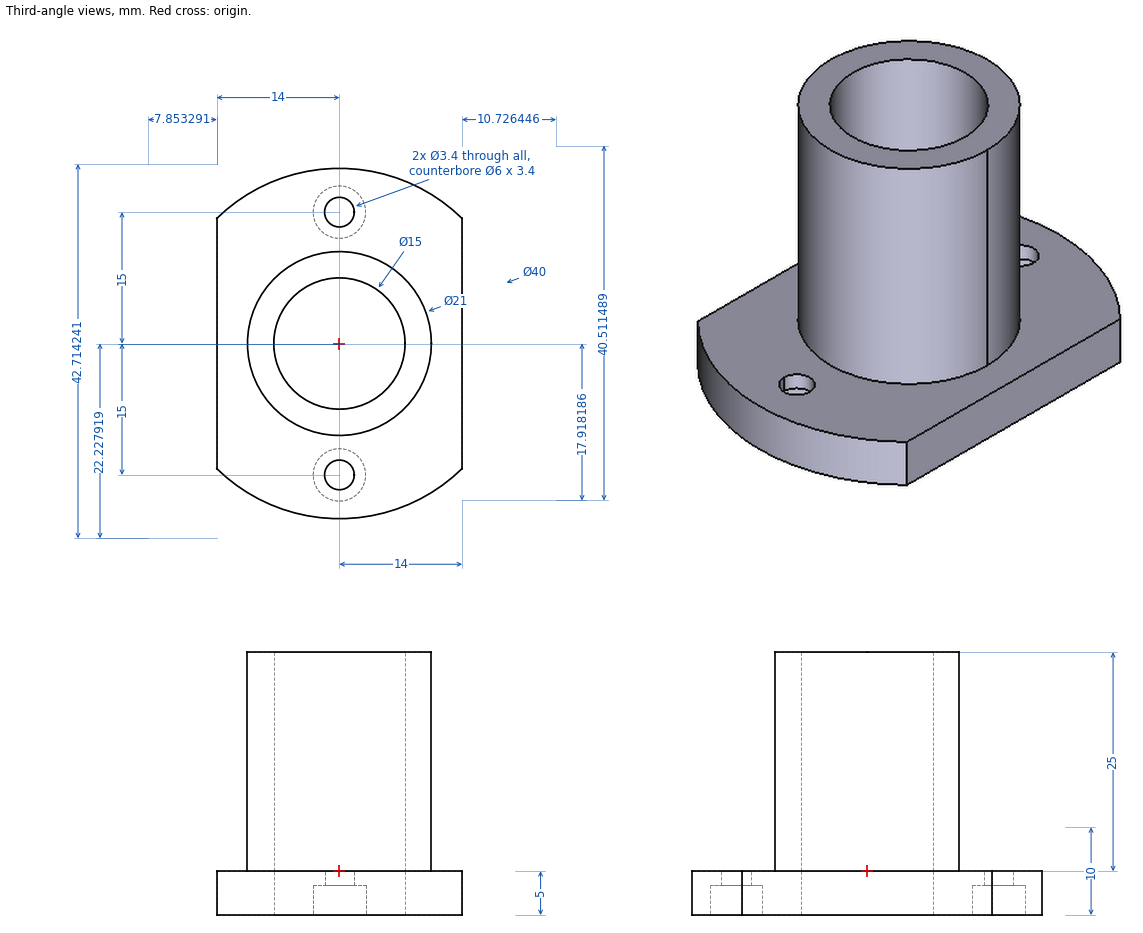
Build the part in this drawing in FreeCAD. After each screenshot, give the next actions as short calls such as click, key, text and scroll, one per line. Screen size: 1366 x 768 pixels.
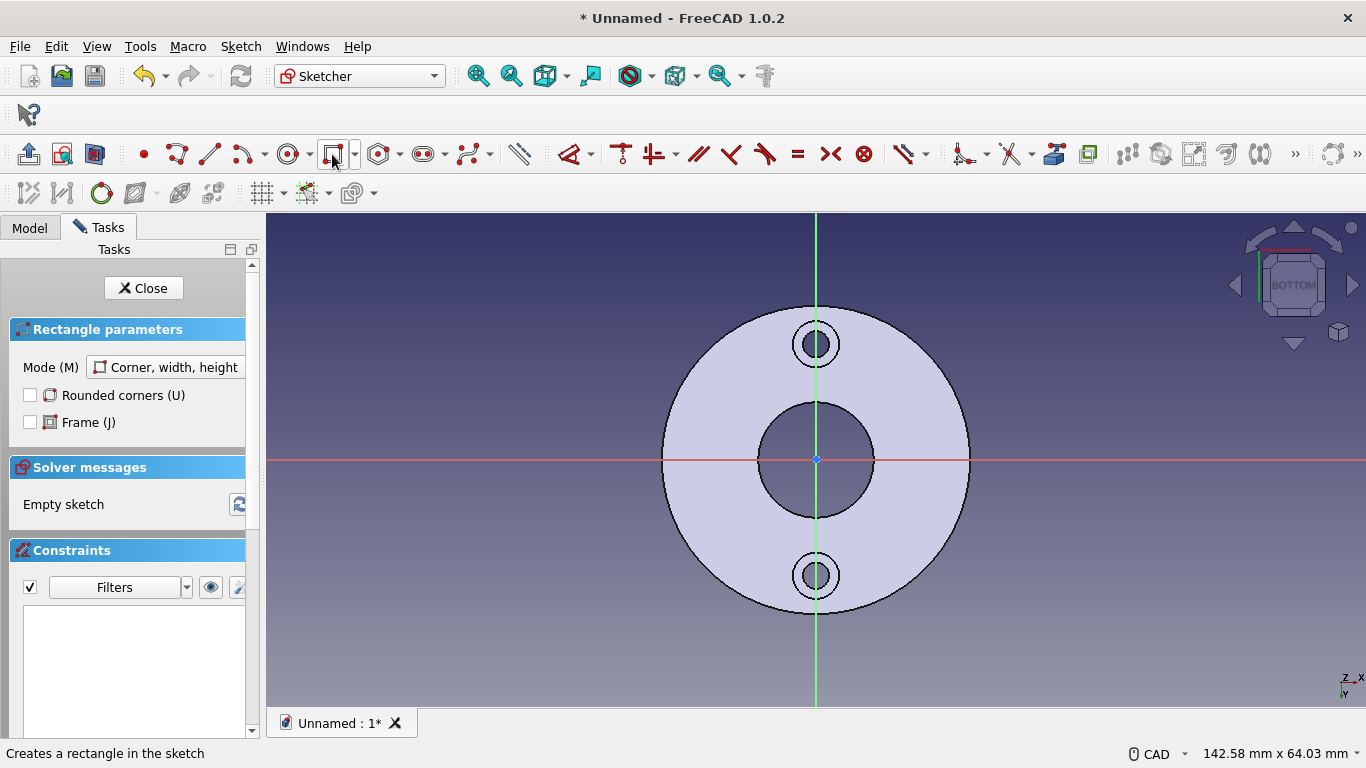
click(924, 322)
move(1007, 634)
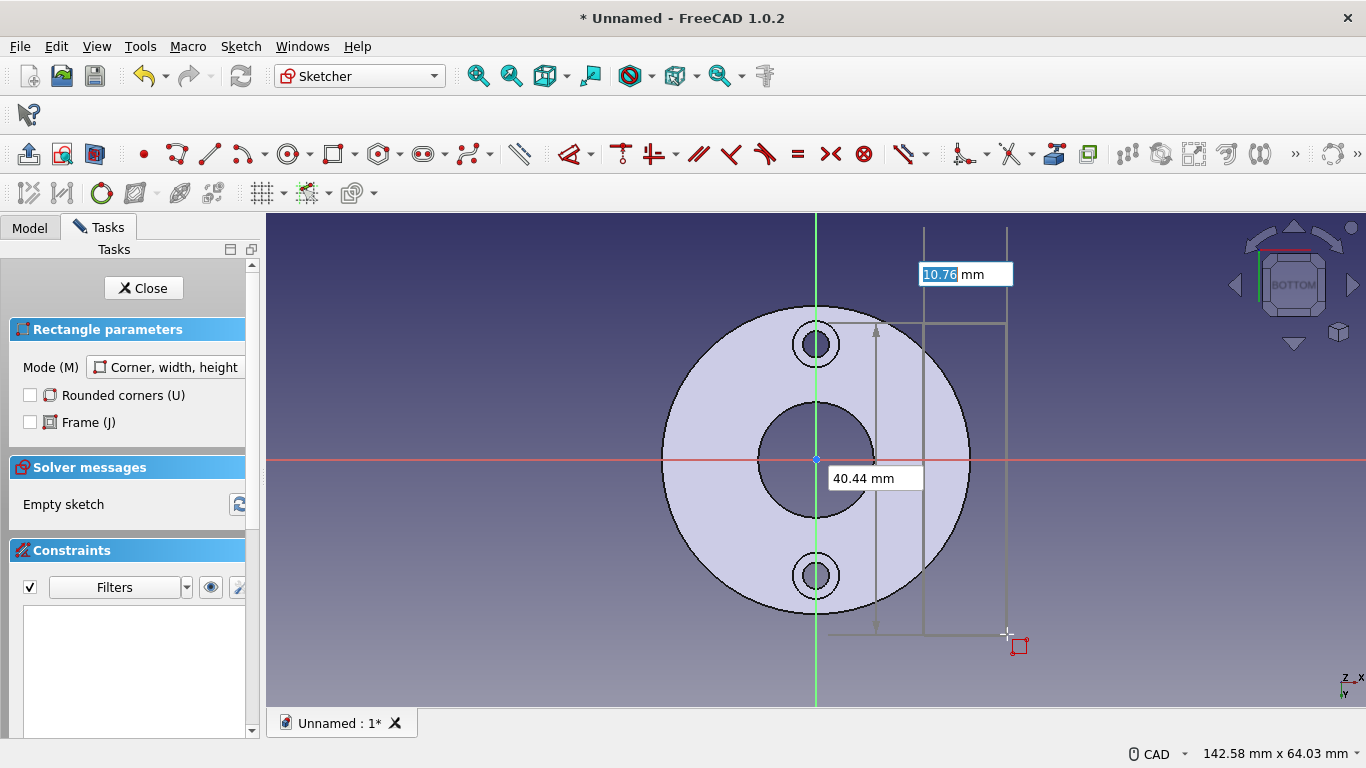
text(10.726446)
key(Tab)
text(40.511489)
key(Return)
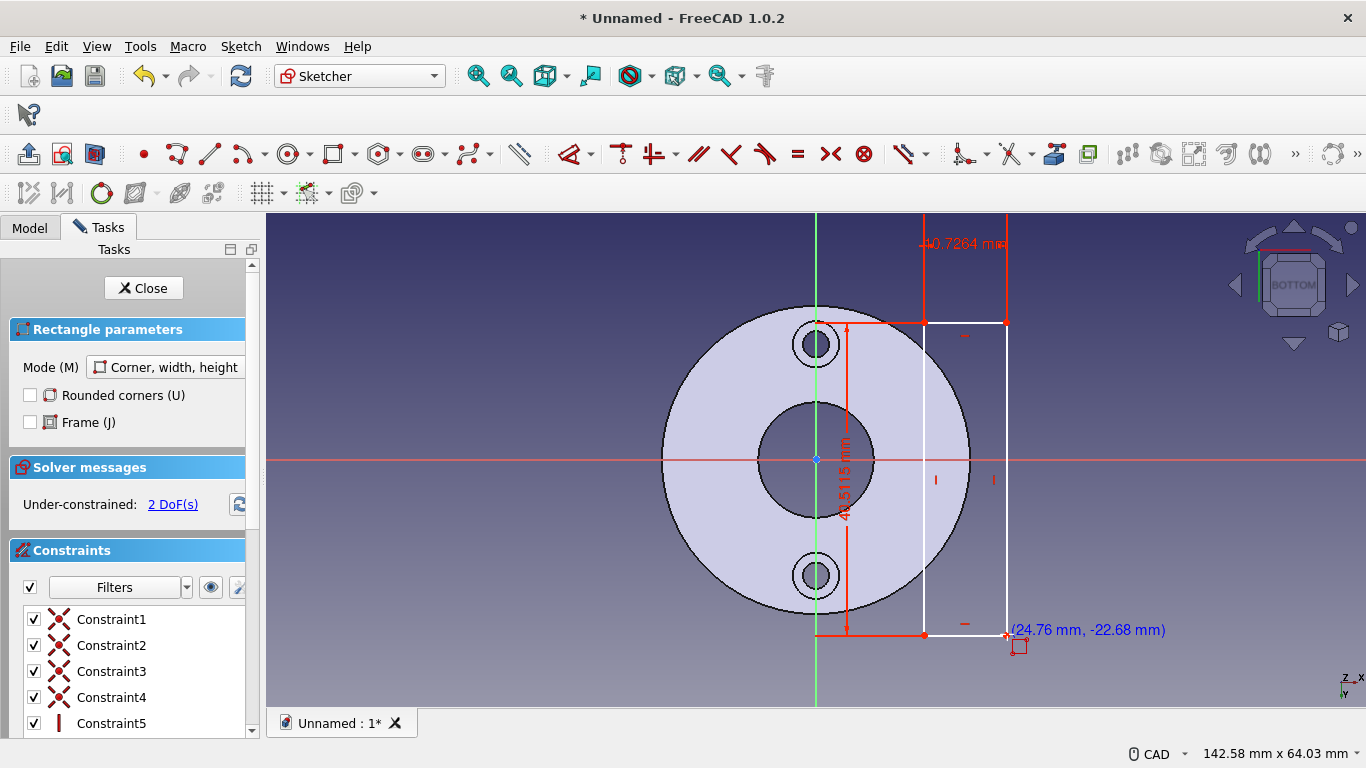
click(647, 289)
move(708, 618)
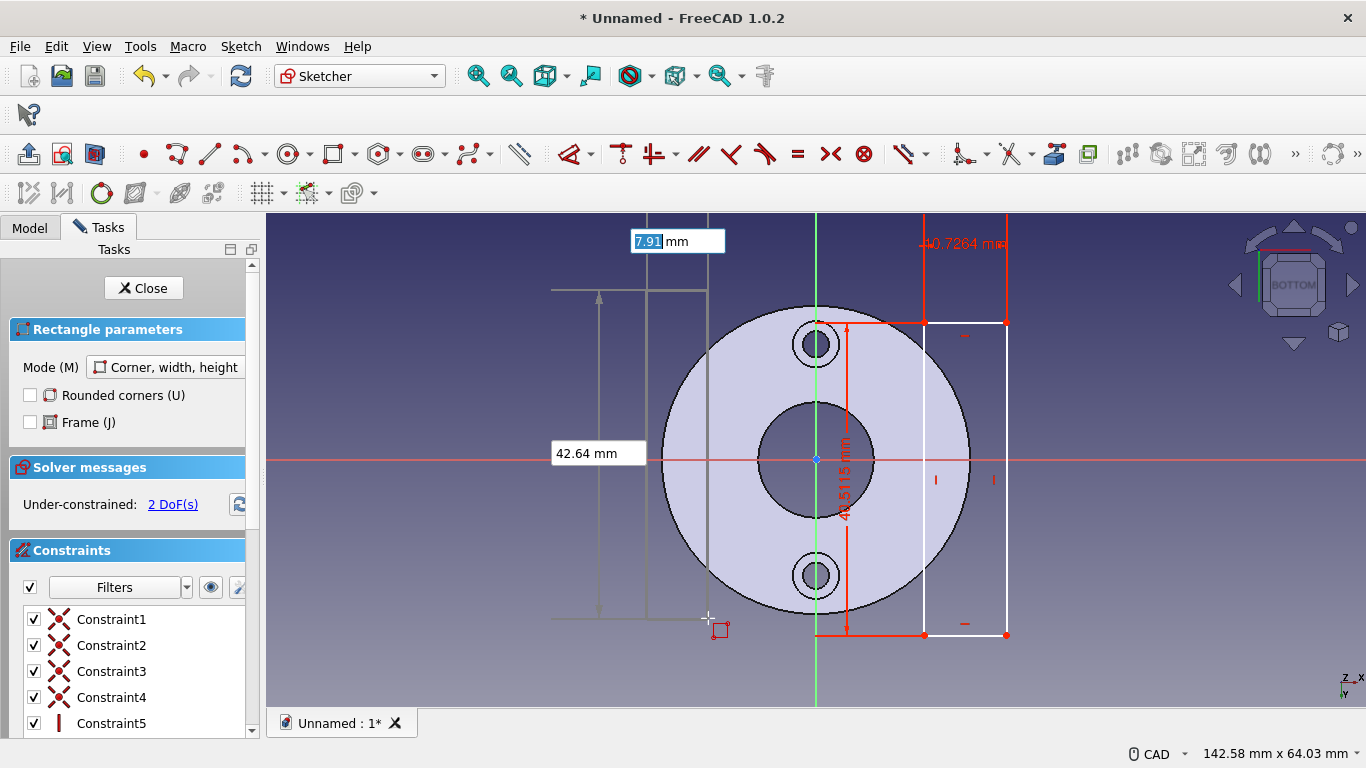
text(7.853291)
key(Tab)
text(42.714241)
key(Return)
key(Escape)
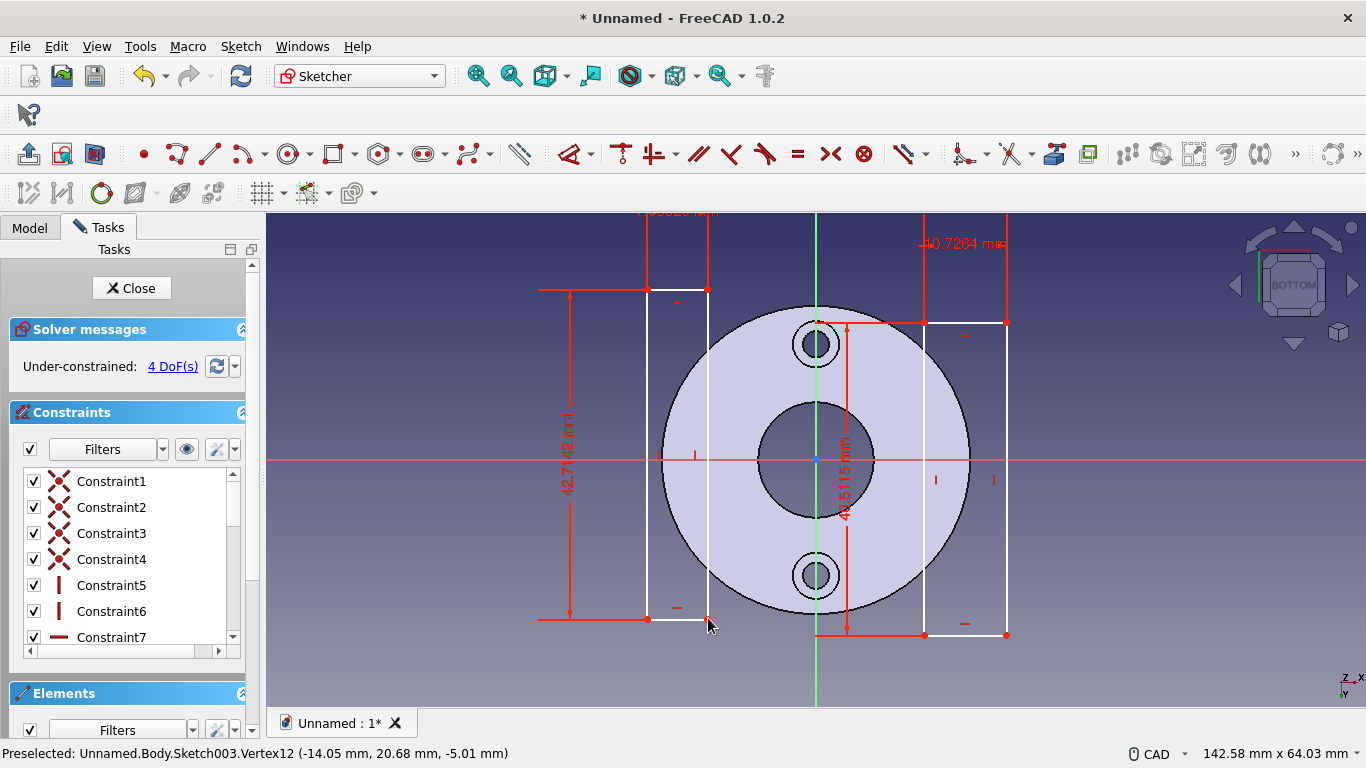
click(568, 154)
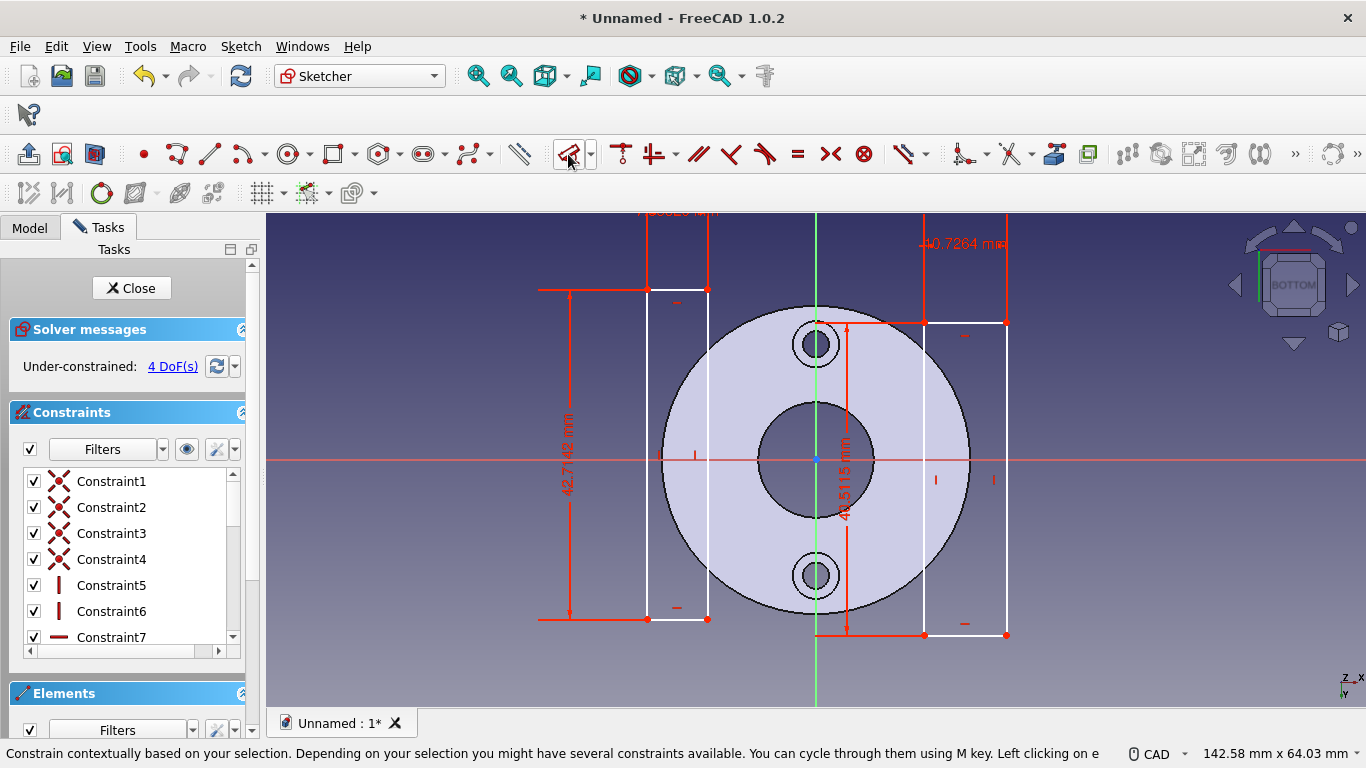
click(924, 323)
click(870, 289)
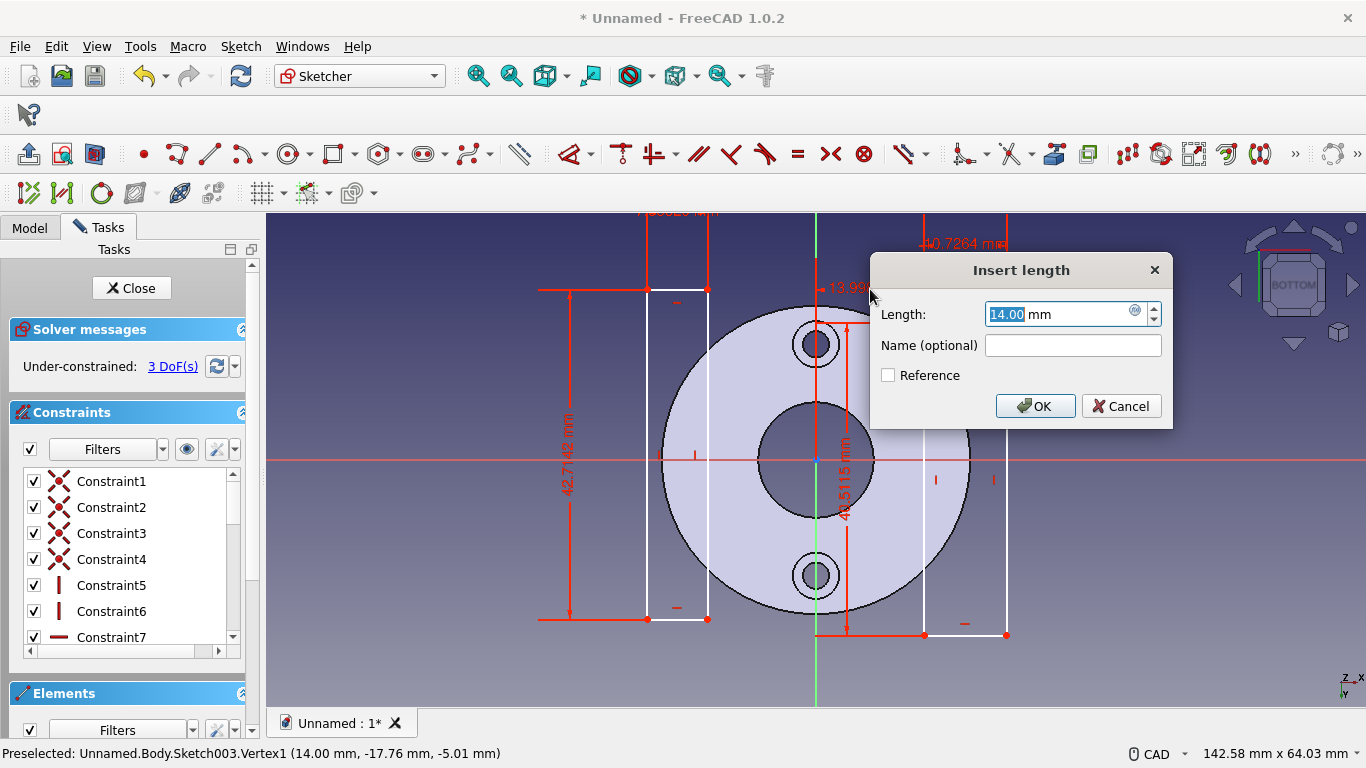
text(14)
key(Return)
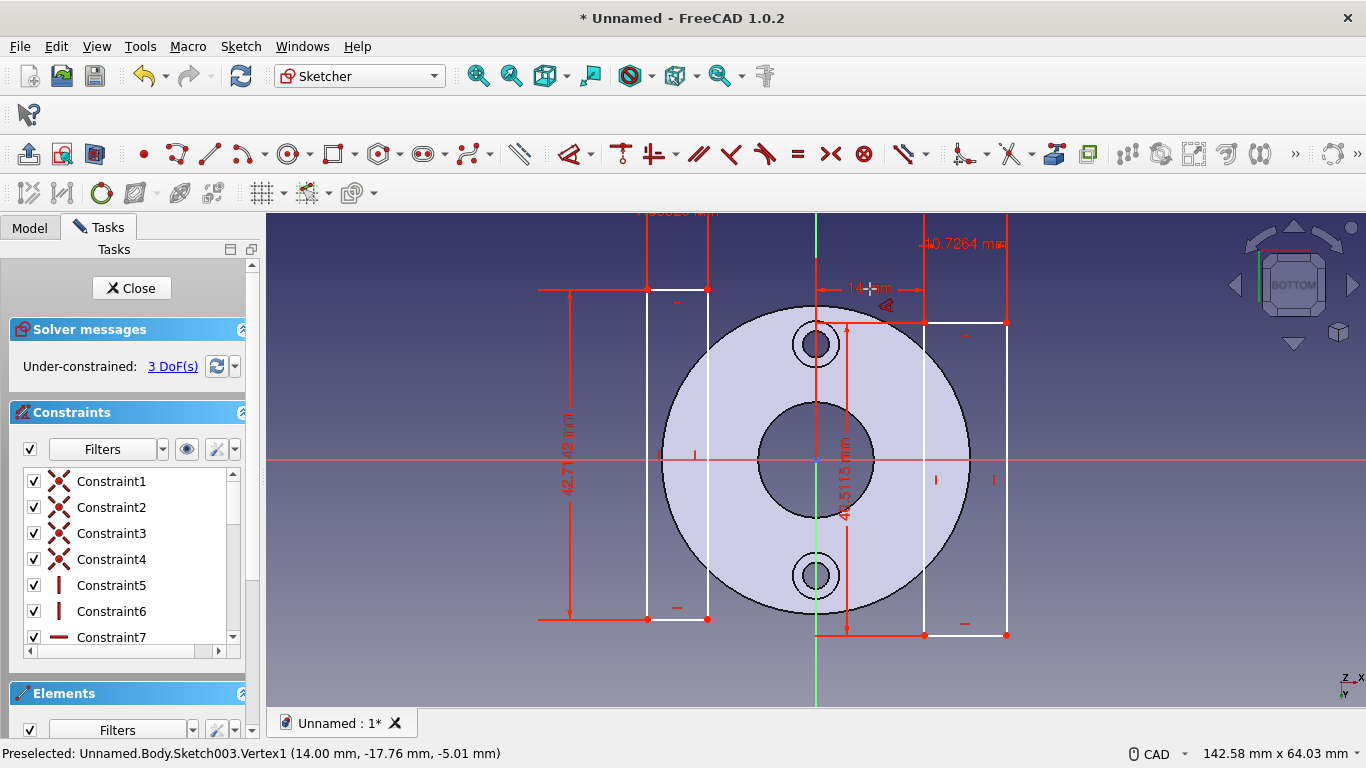
click(708, 620)
click(762, 654)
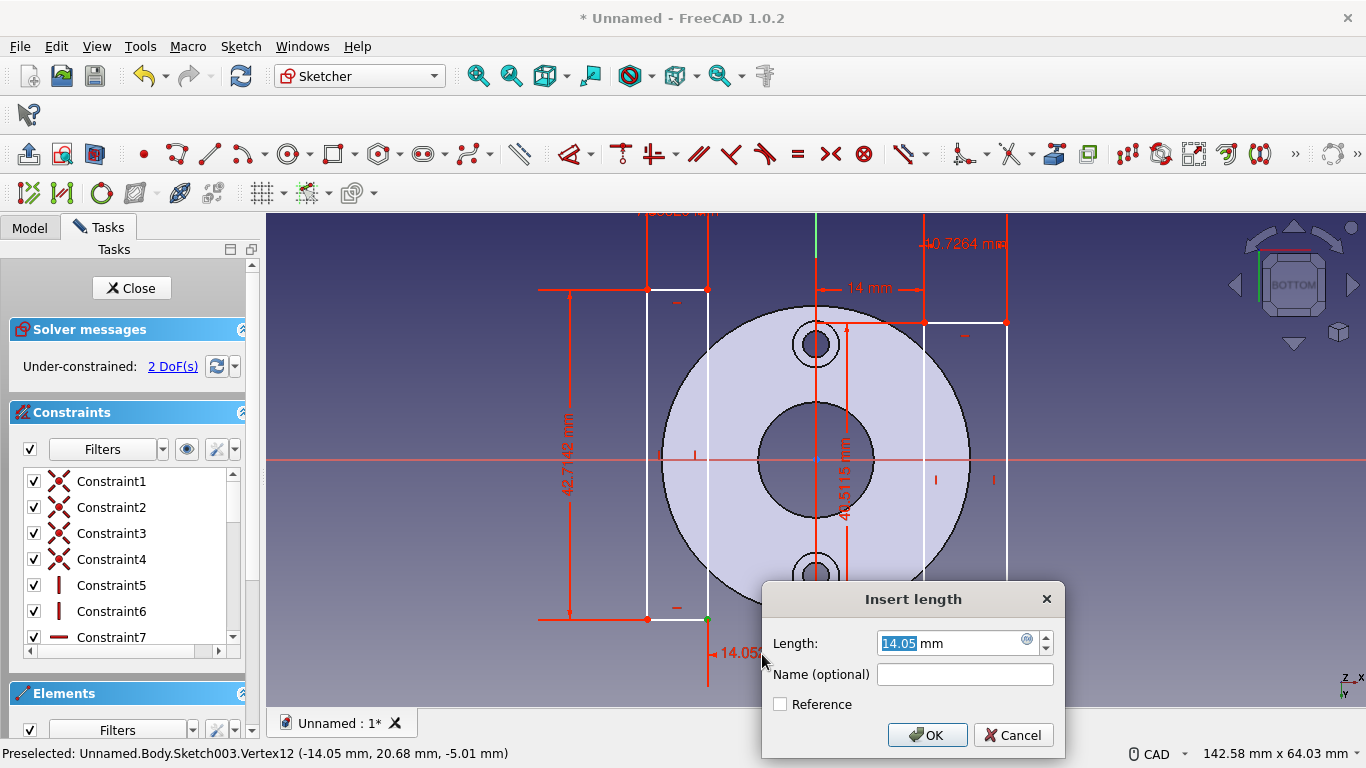
text(14)
key(Return)